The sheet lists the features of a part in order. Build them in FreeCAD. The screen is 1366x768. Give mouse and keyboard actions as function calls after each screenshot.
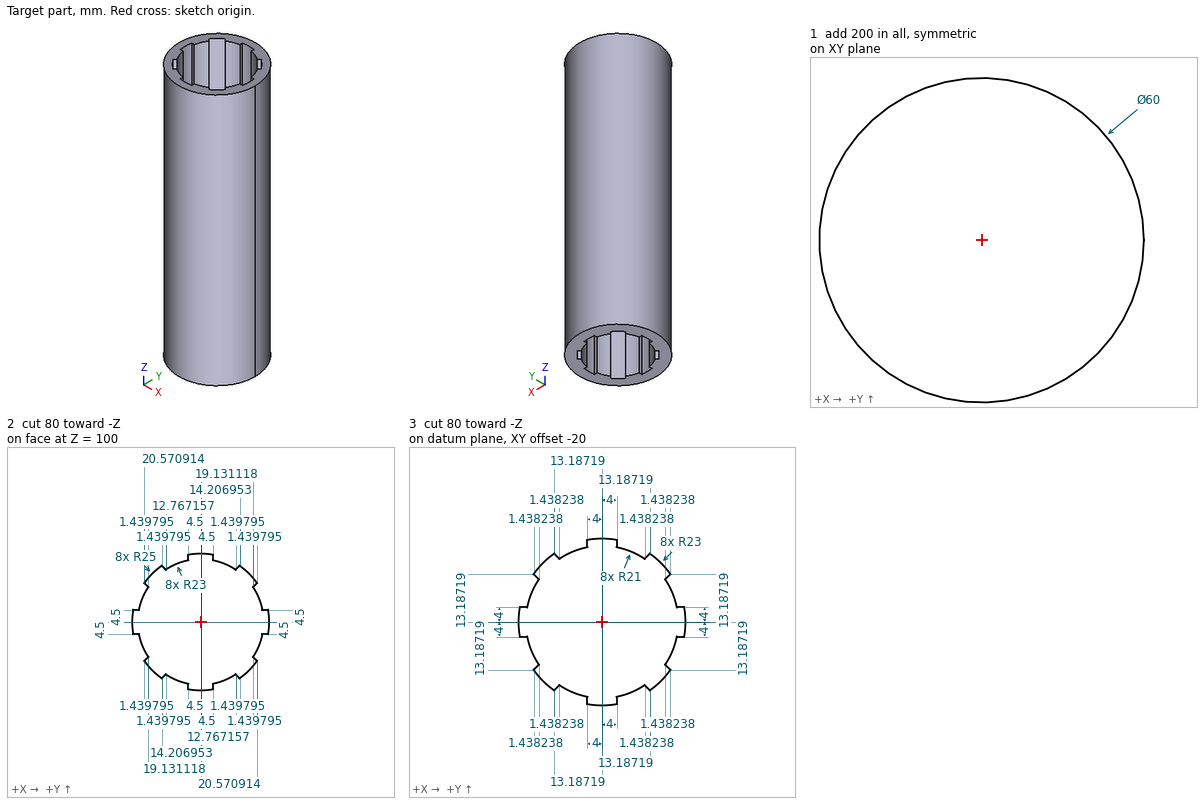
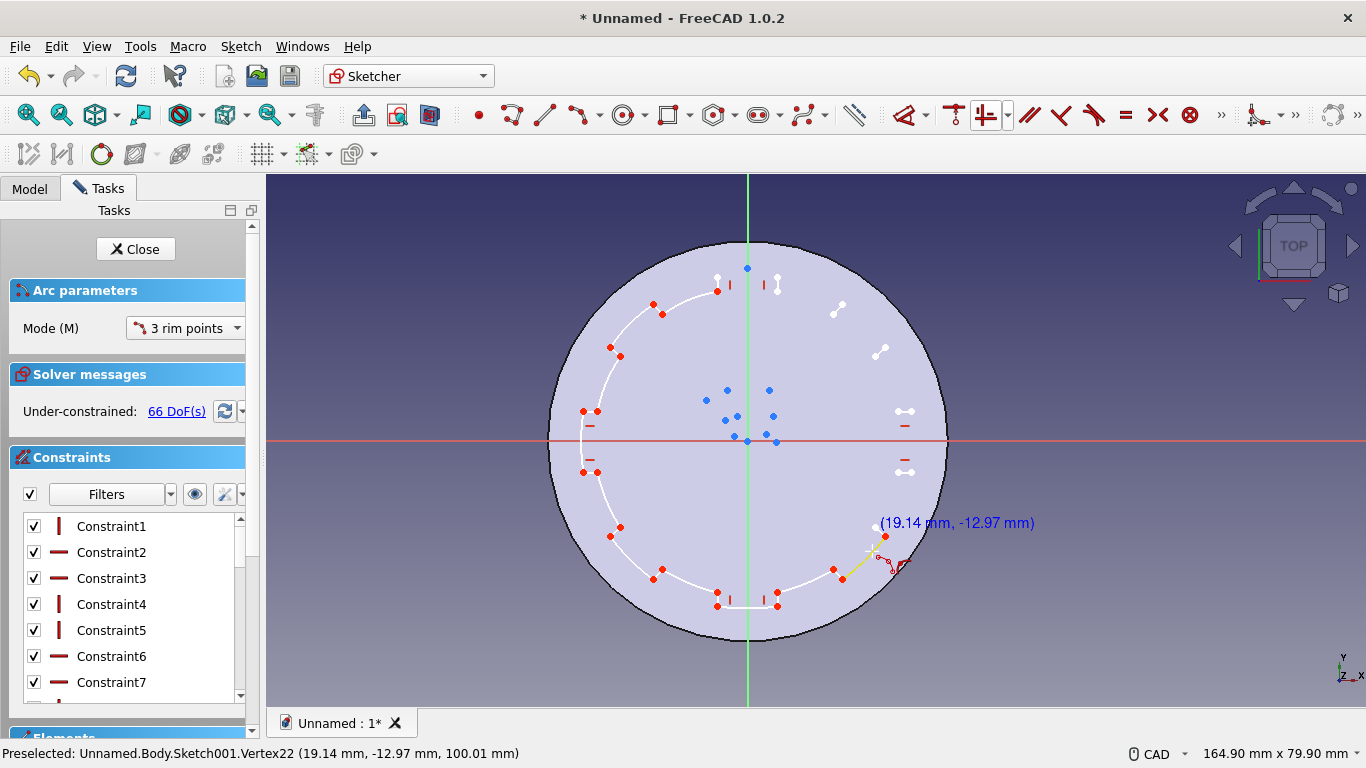
scroll(898, 471, up, 5)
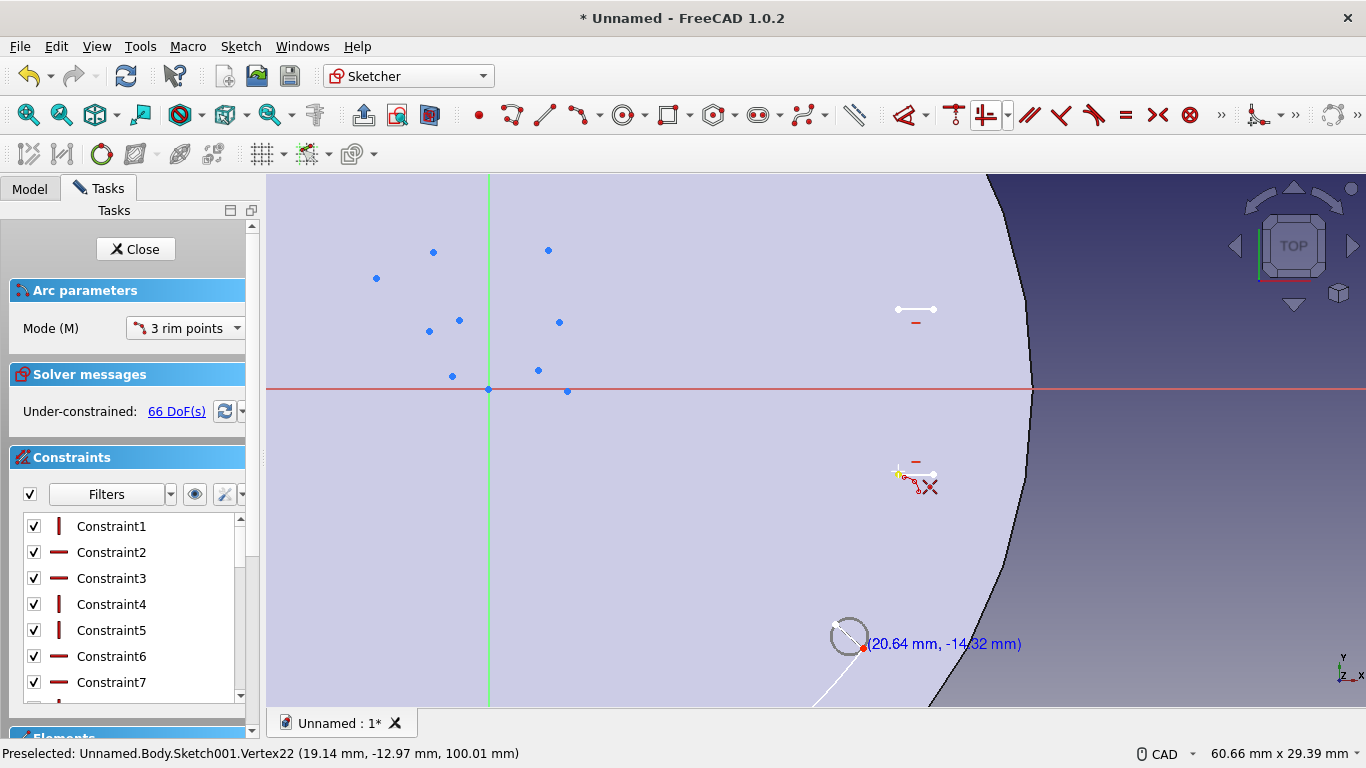
click(898, 475)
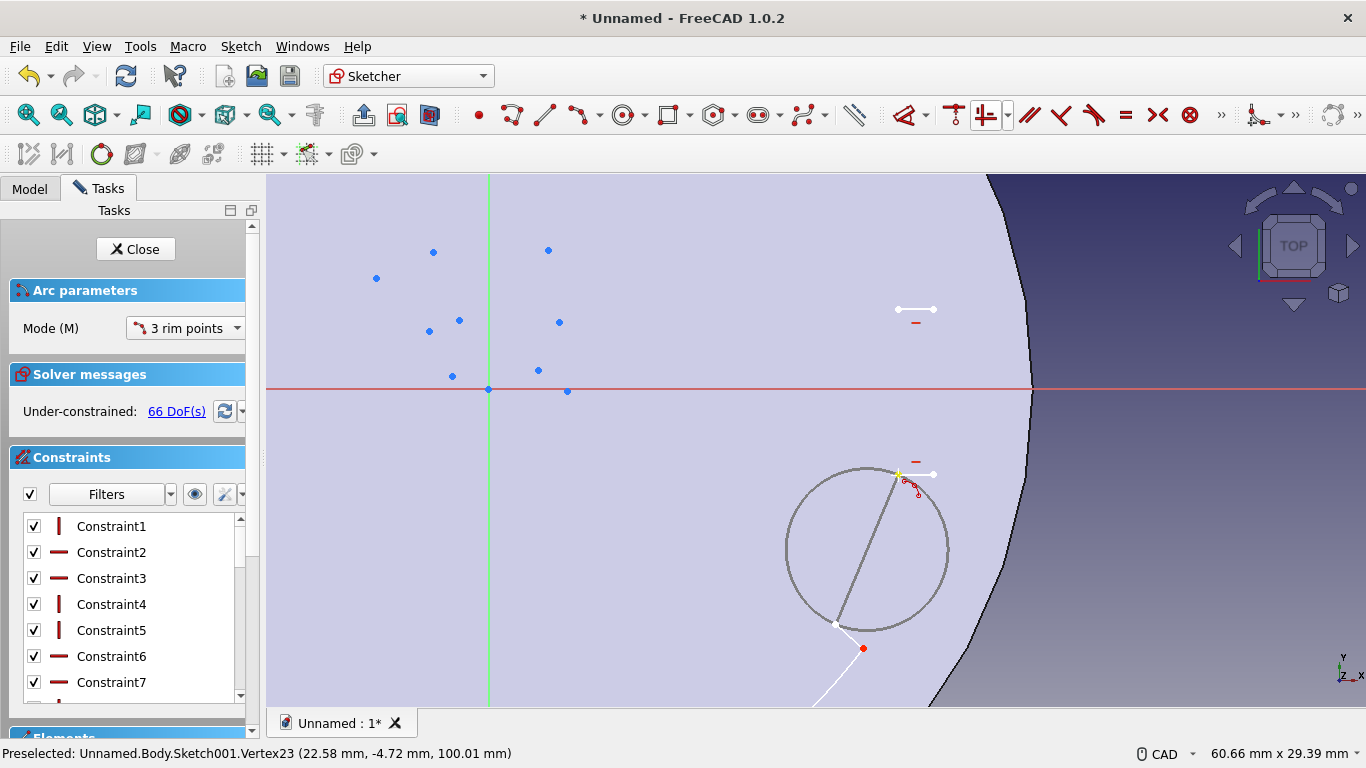
scroll(874, 549, up, 4)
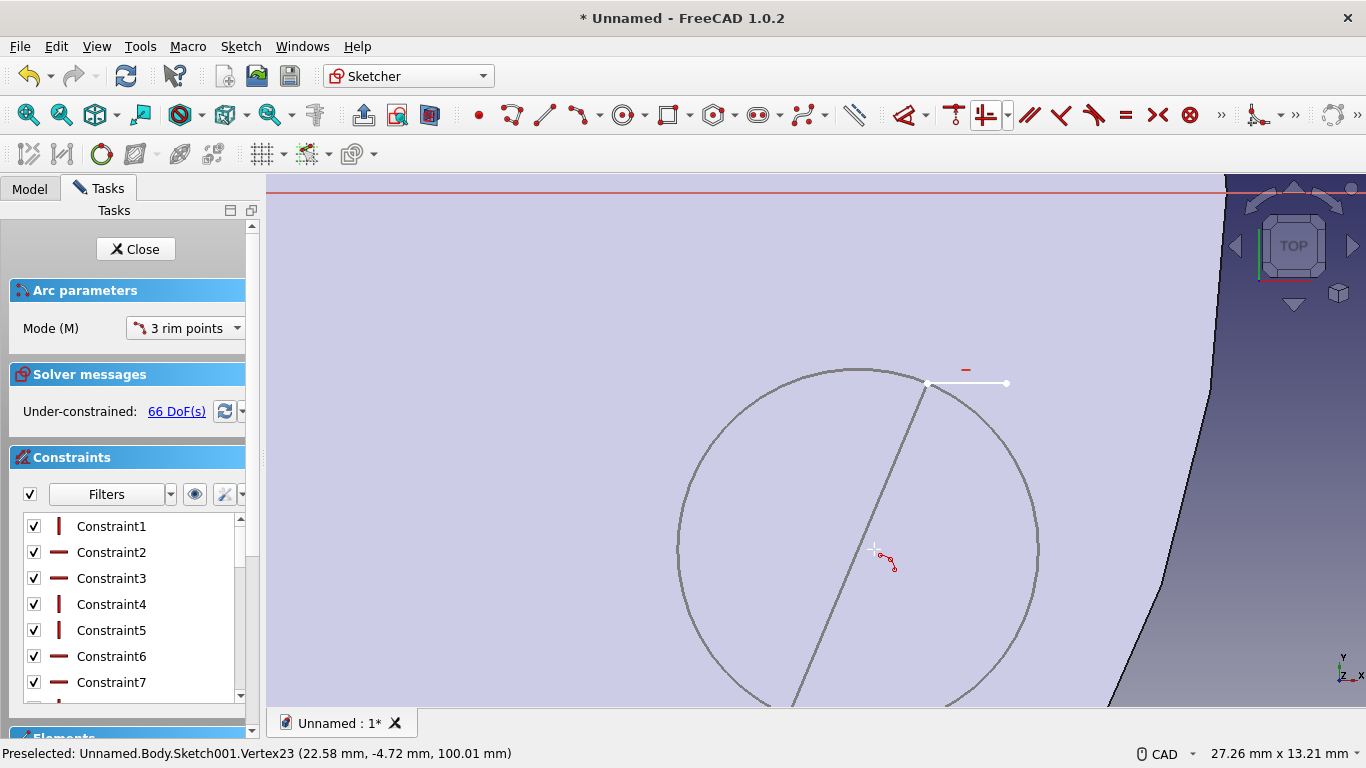
click(874, 548)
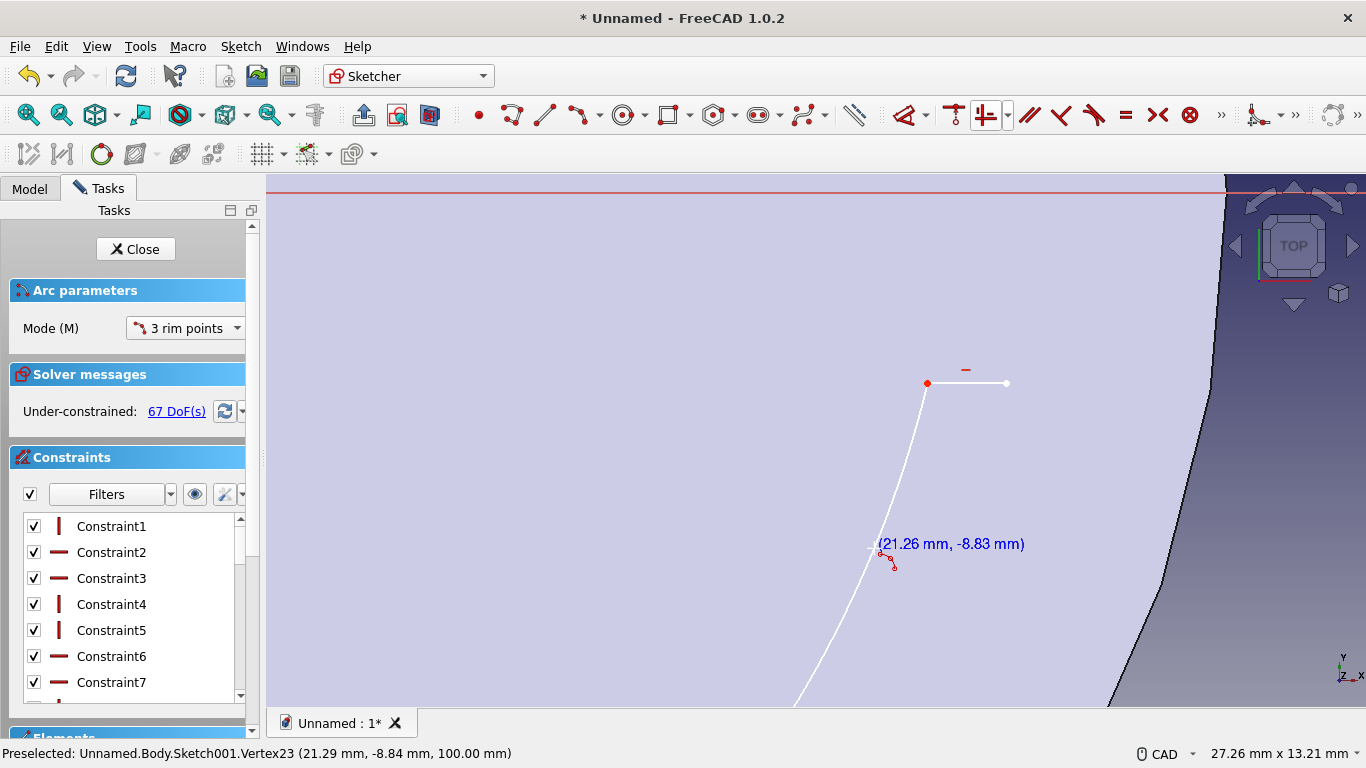
click(1006, 383)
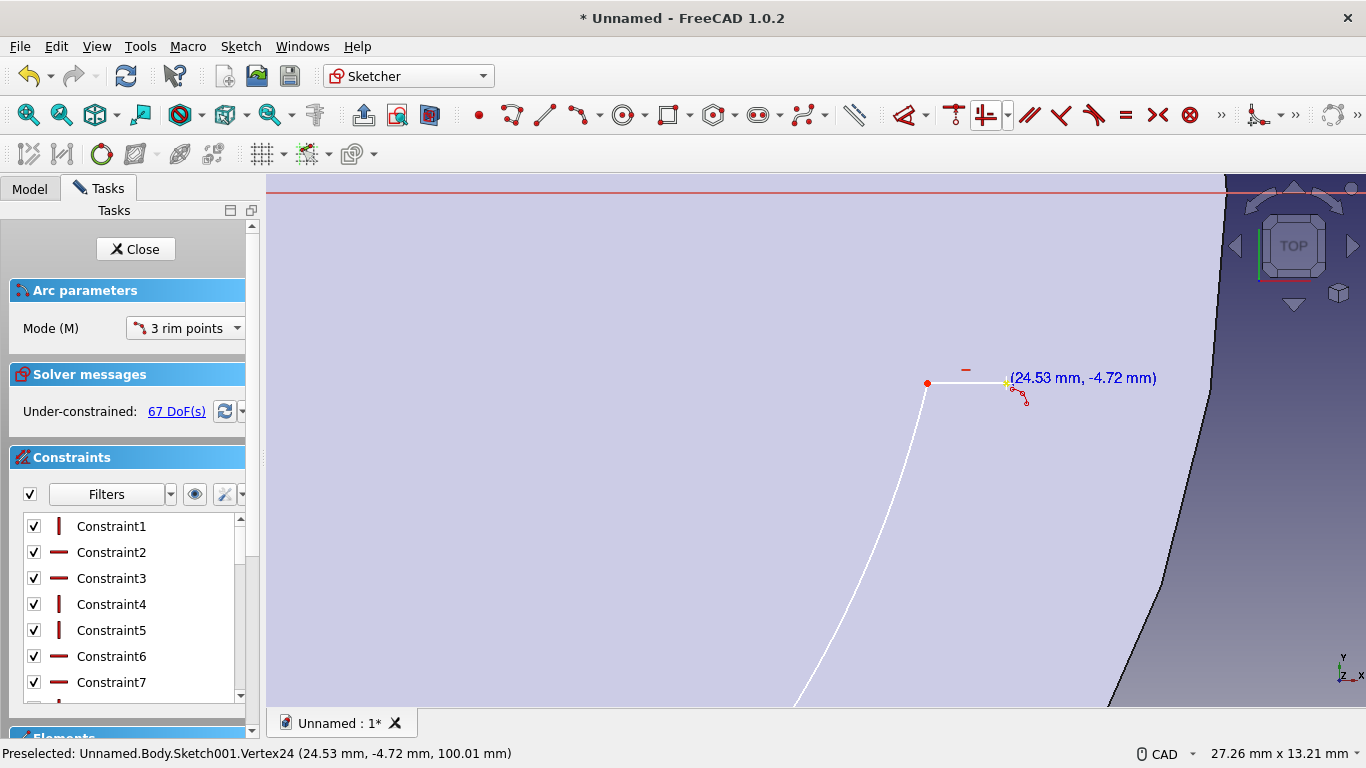
scroll(892, 490, down, 9)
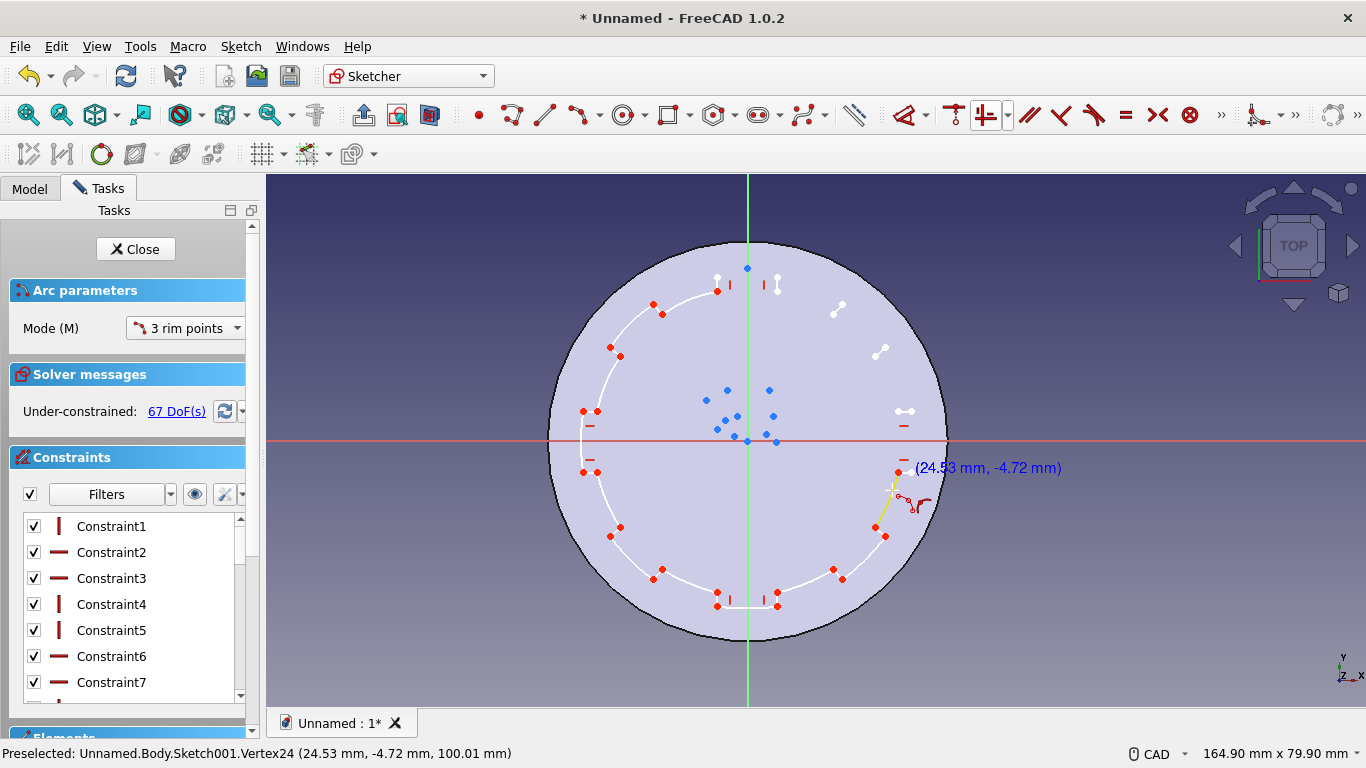
scroll(912, 411, up, 5)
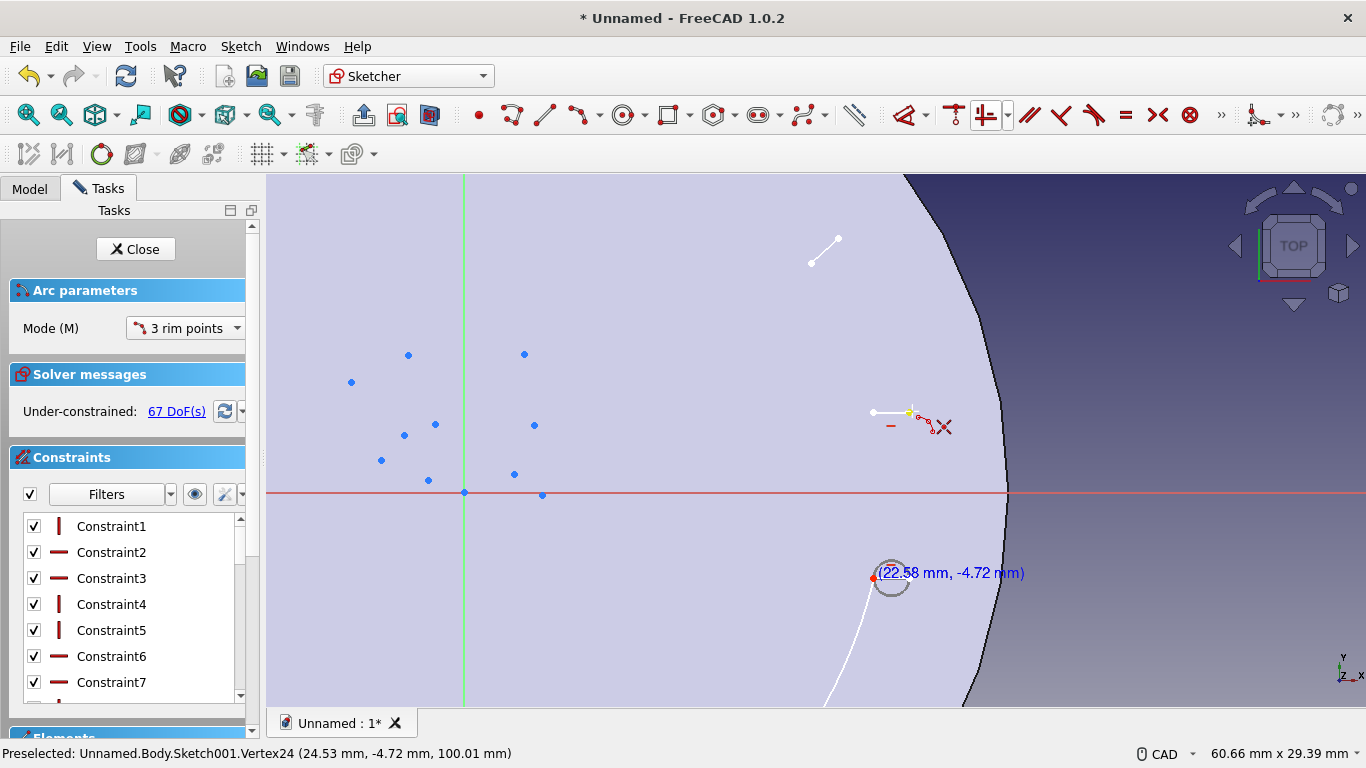
click(909, 413)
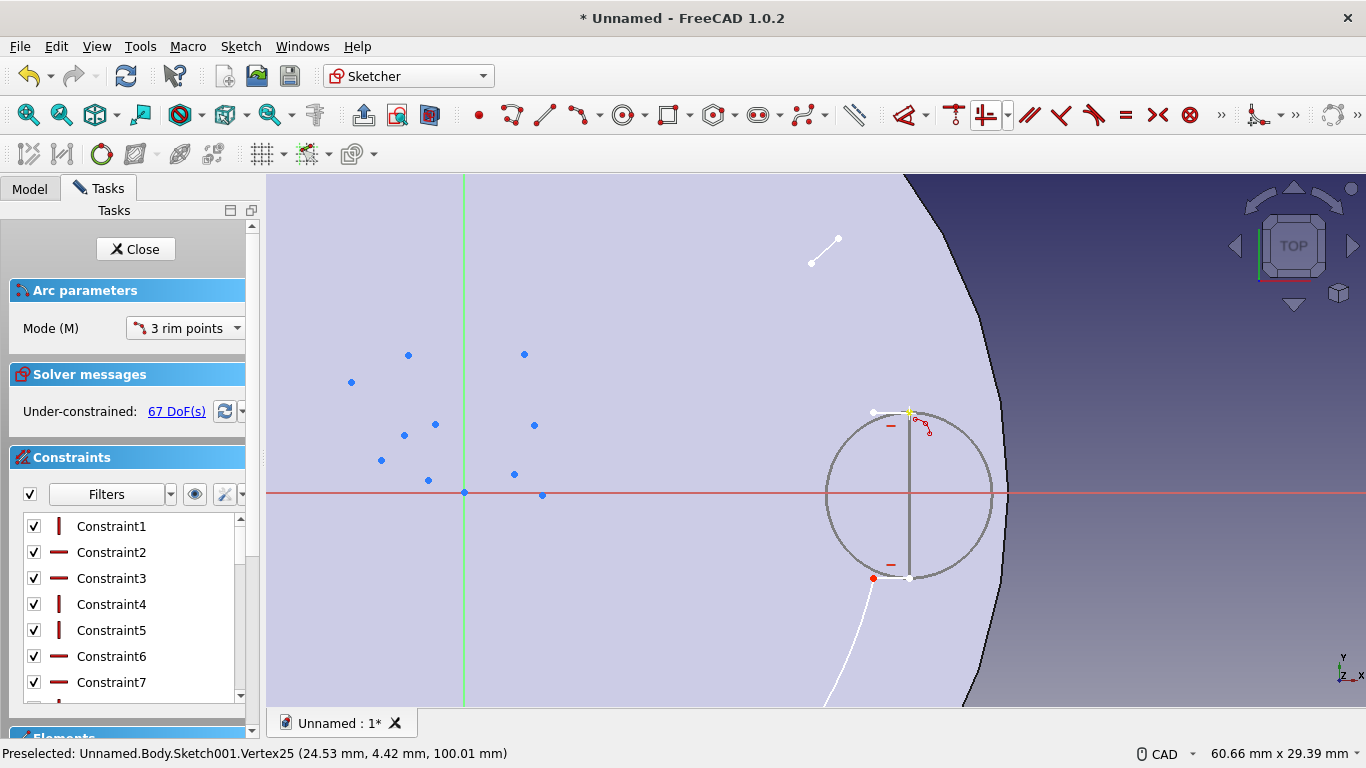
scroll(917, 509, up, 5)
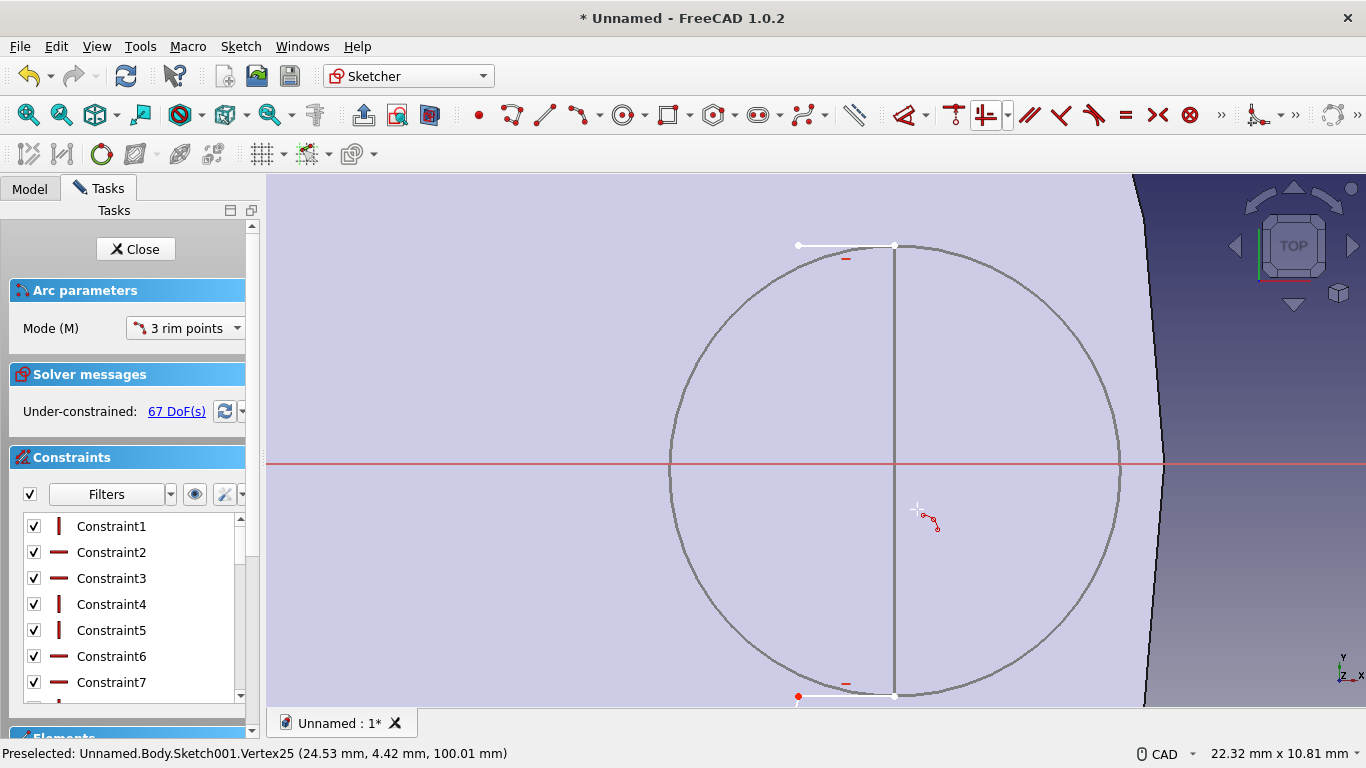
click(917, 508)